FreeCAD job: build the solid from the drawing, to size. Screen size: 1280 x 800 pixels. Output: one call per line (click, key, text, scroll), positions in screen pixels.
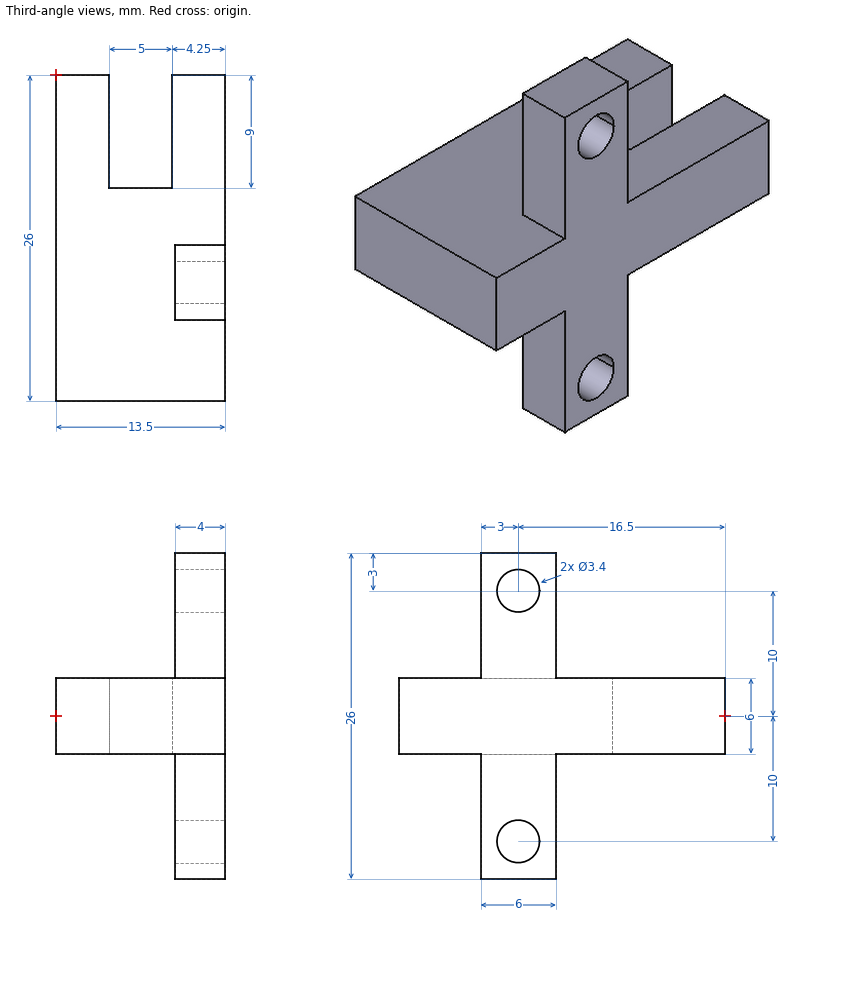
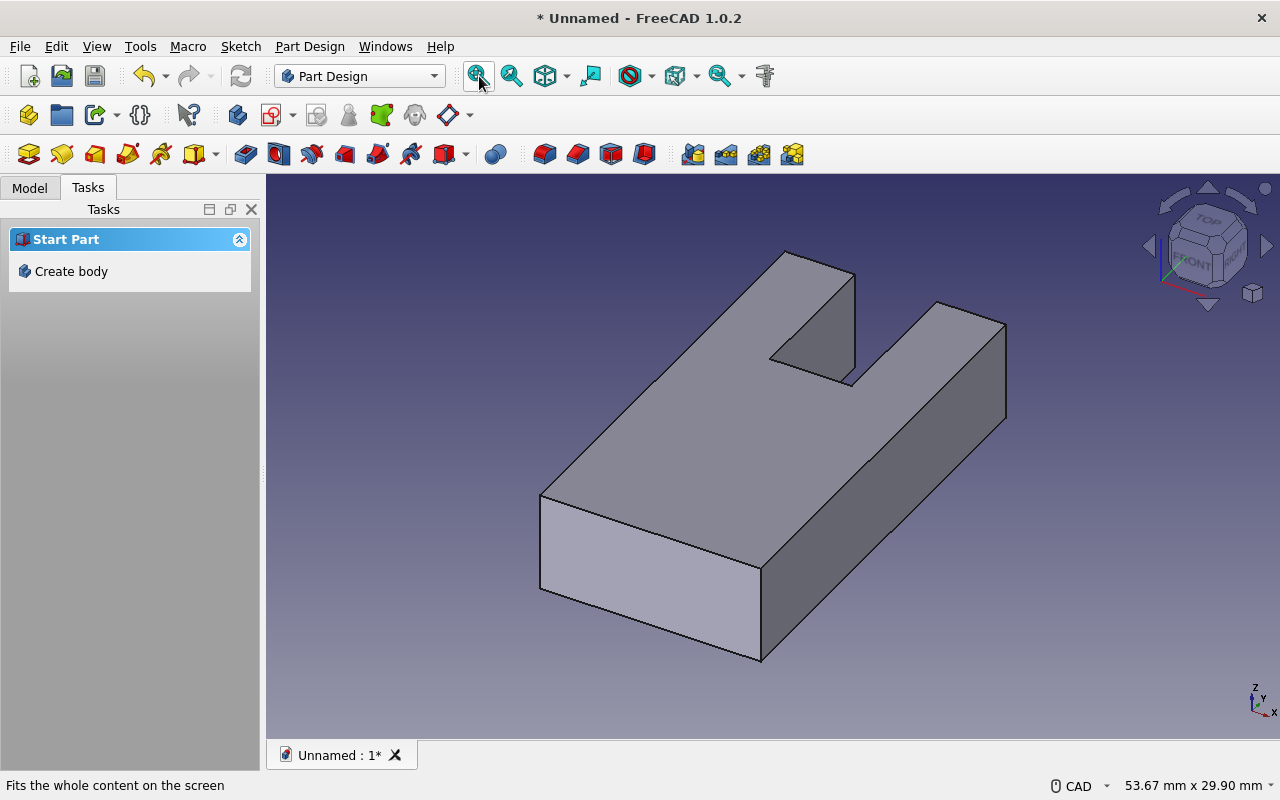
click(954, 422)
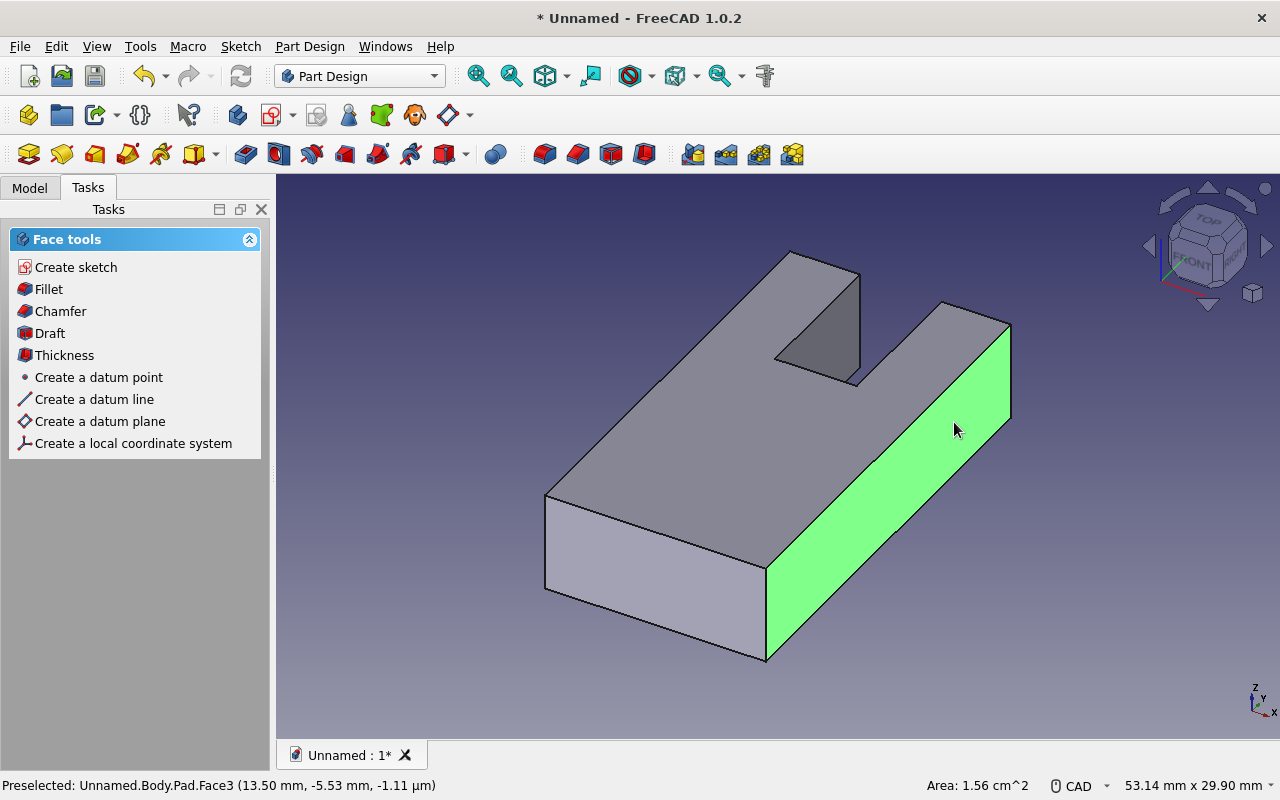
click(270, 116)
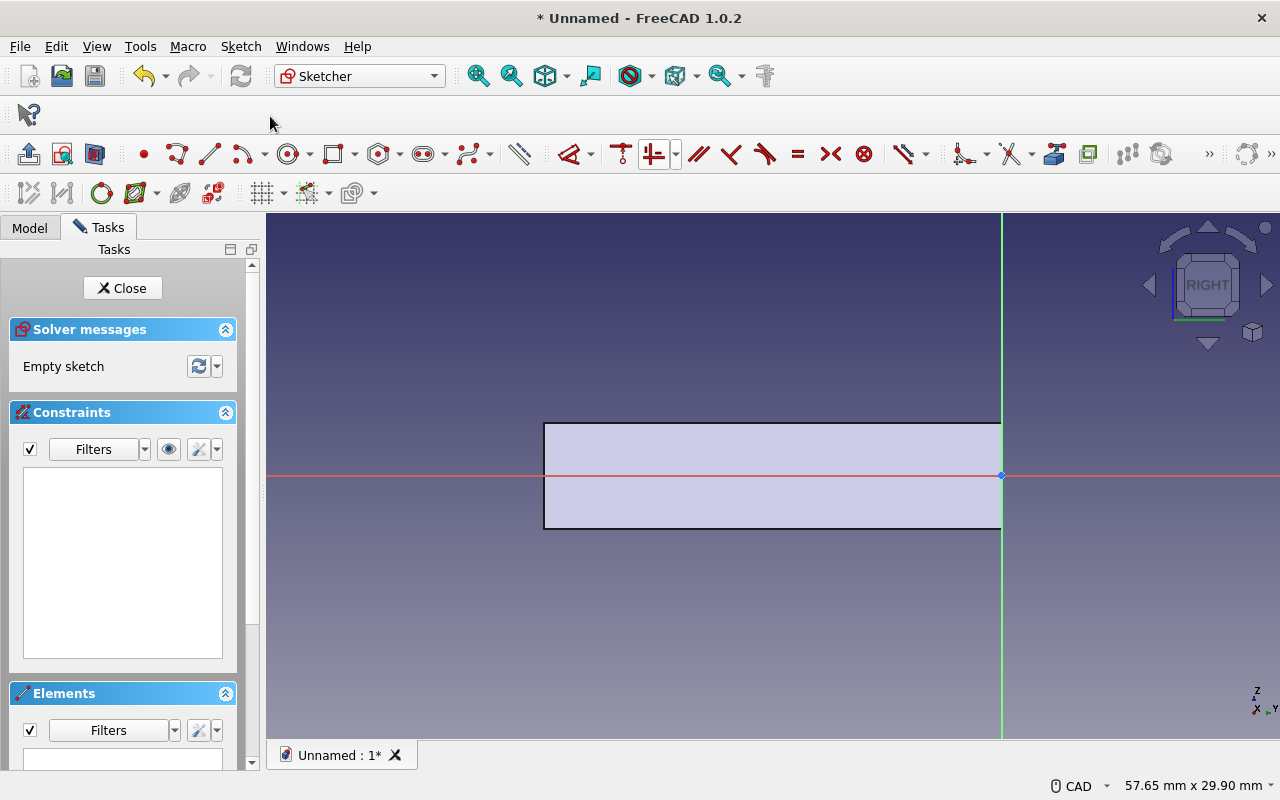
scroll(449, 476, down, 2)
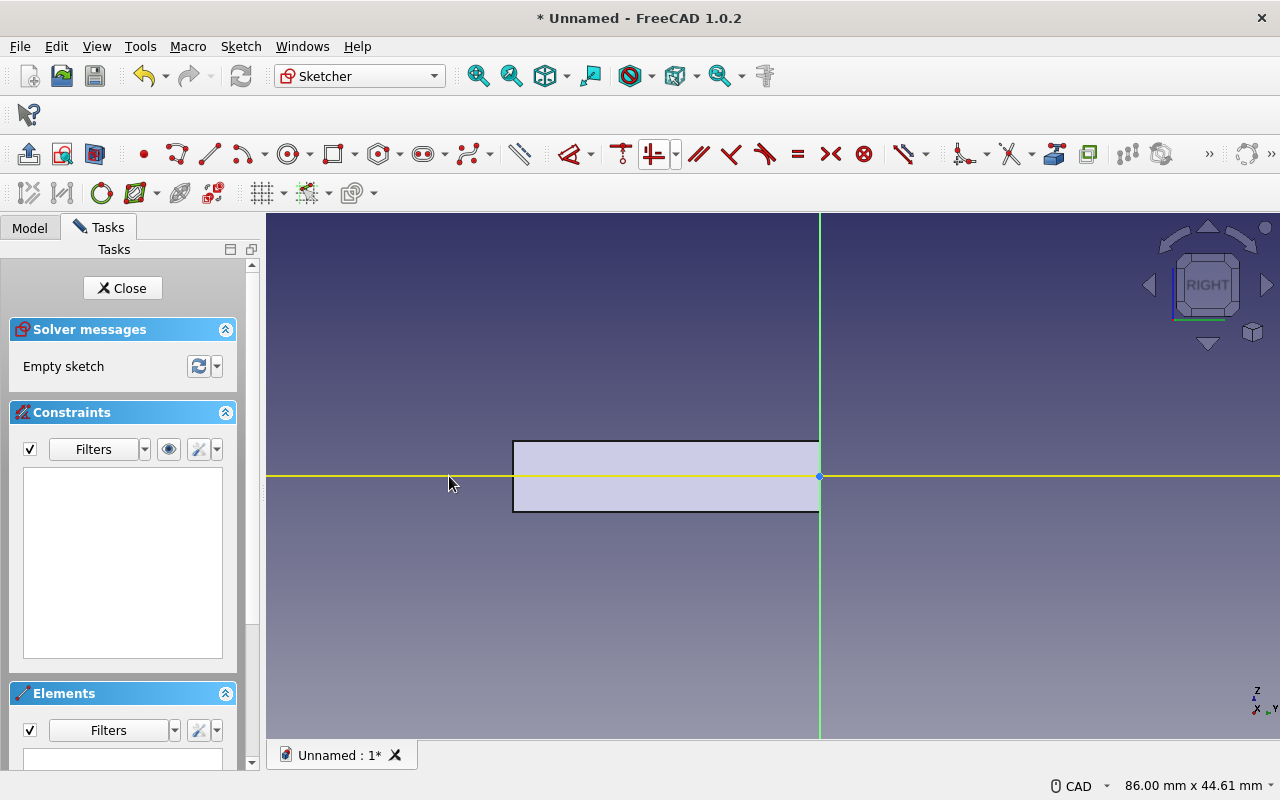
click(332, 154)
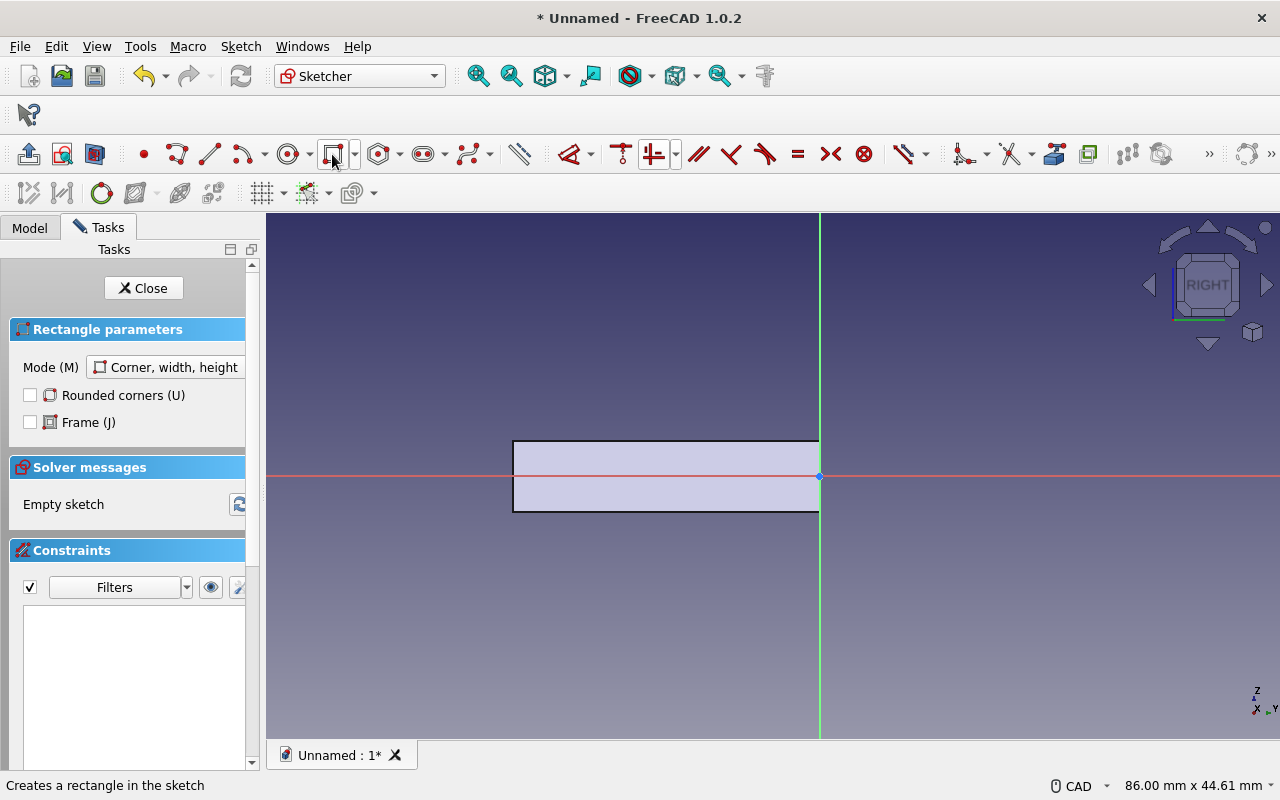
click(590, 323)
move(660, 629)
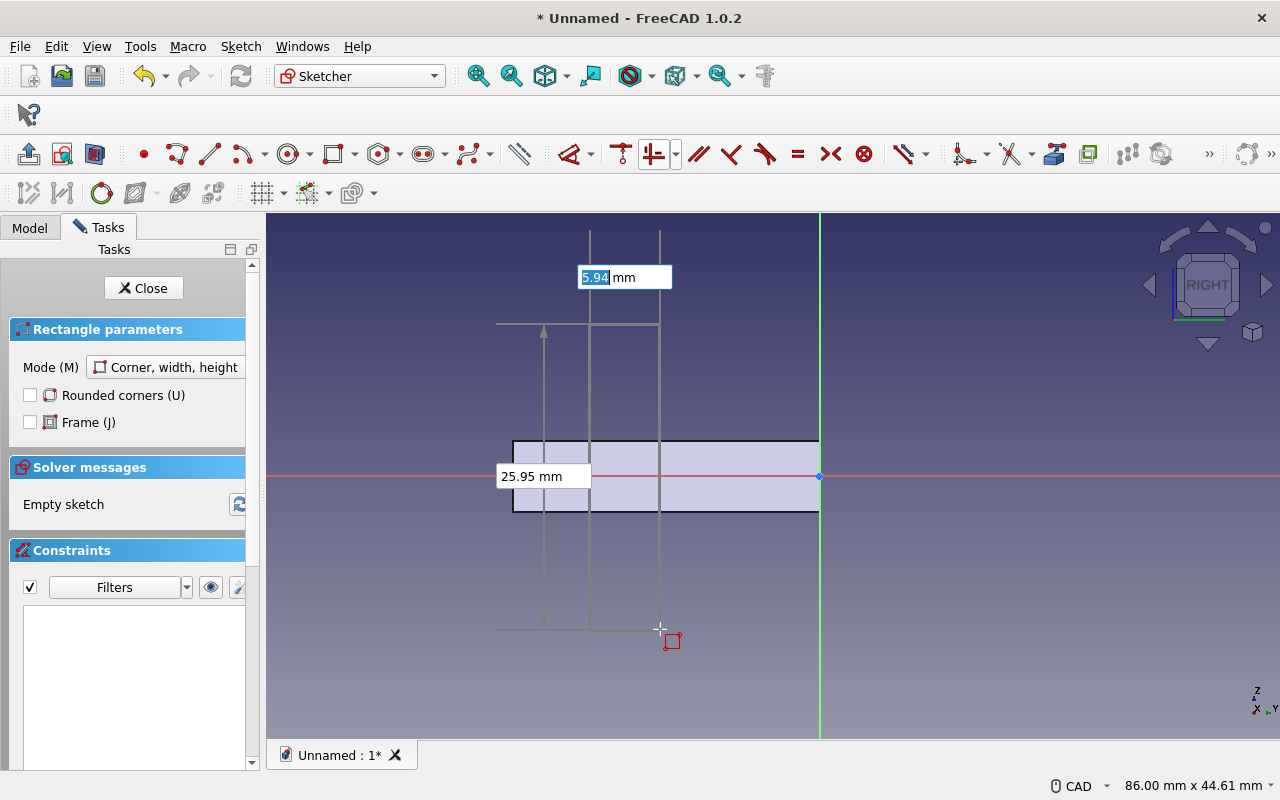
text(6)
key(Tab)
text(26)
key(Return)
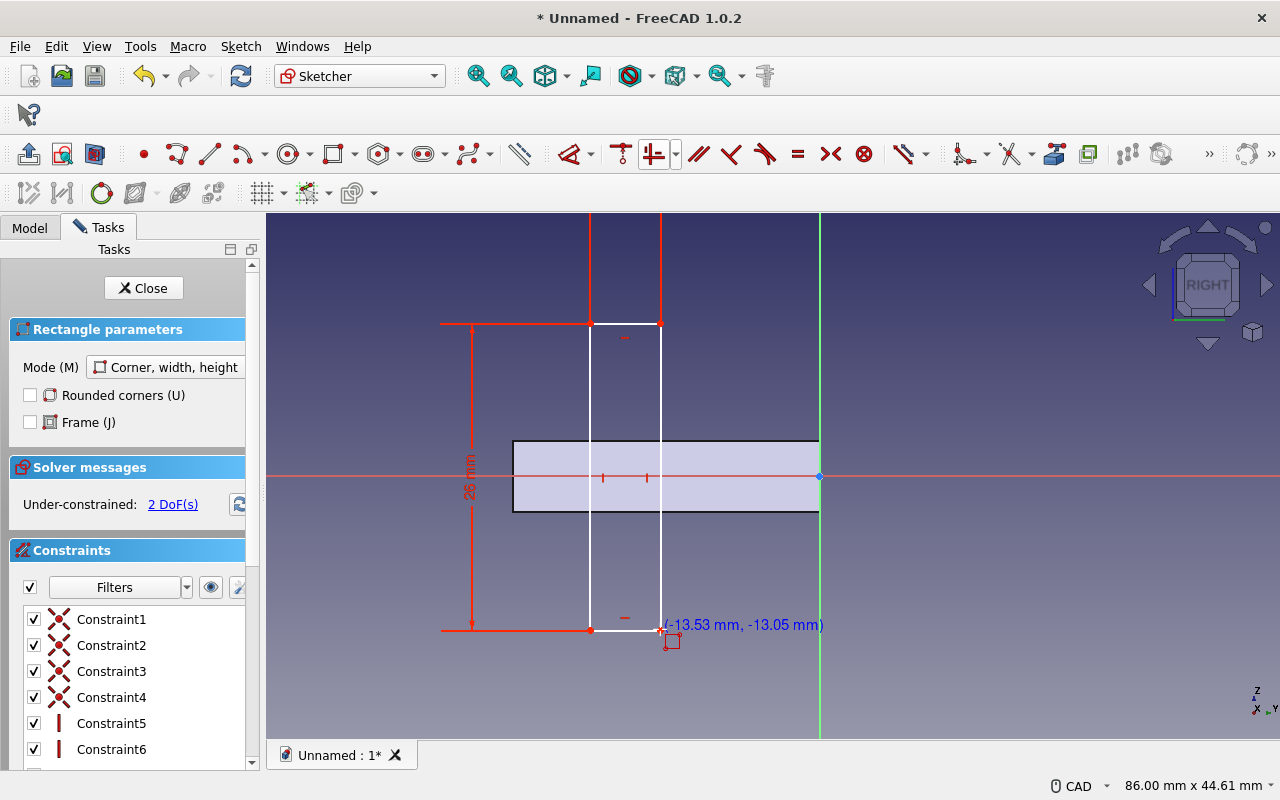
click(288, 154)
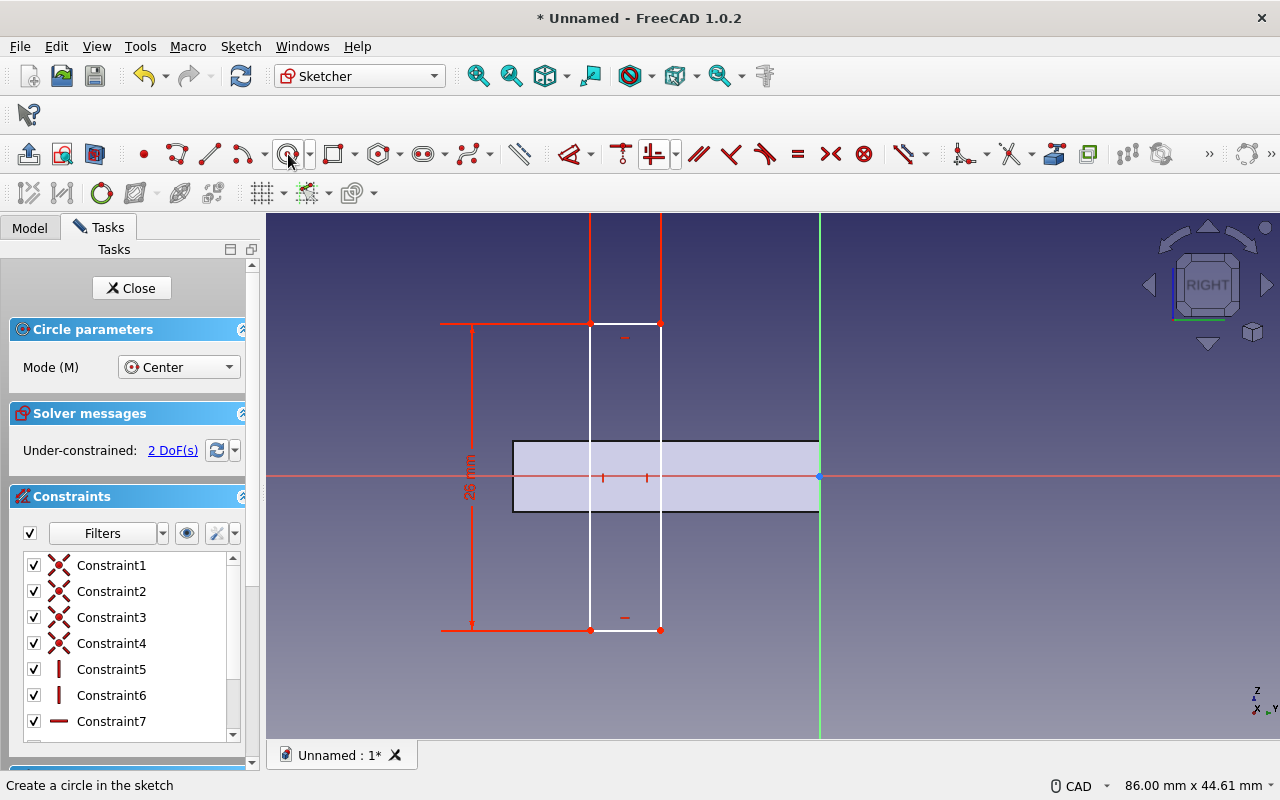
click(625, 358)
move(639, 344)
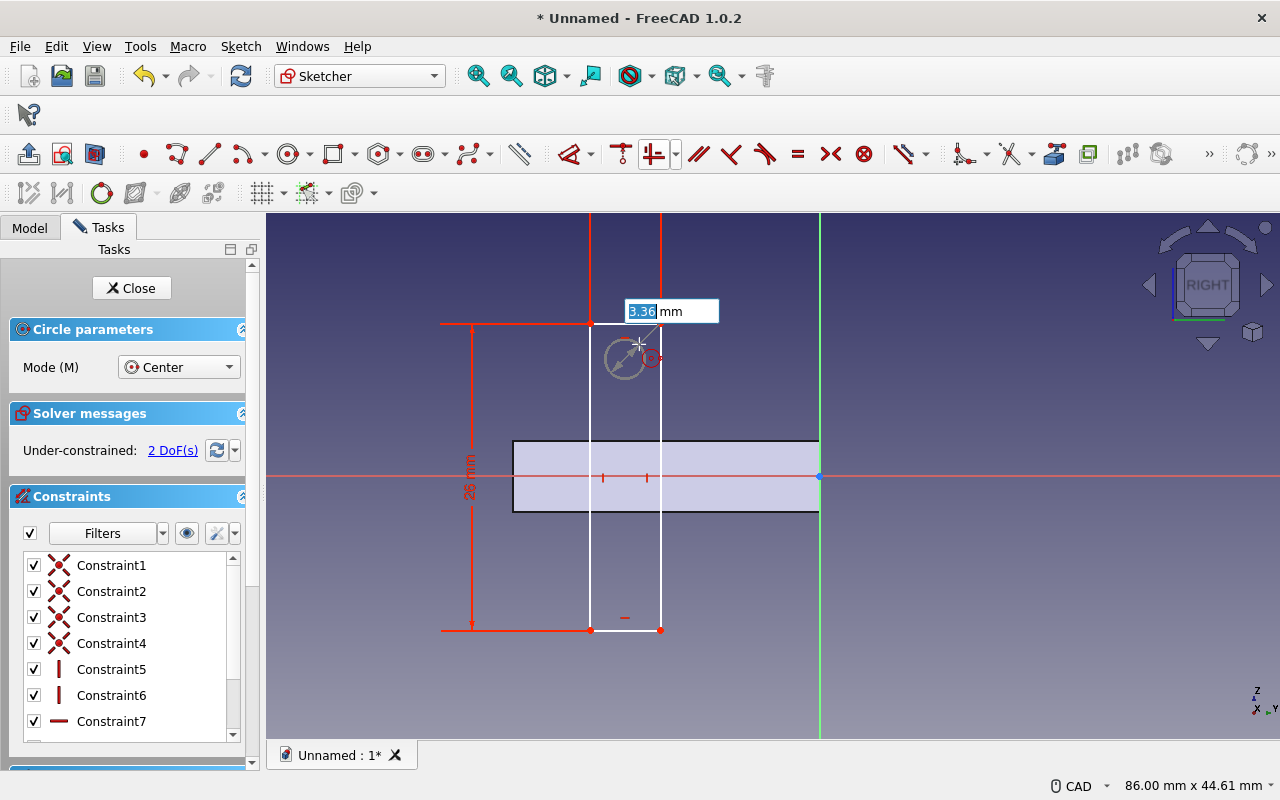
text(3.4)
key(Return)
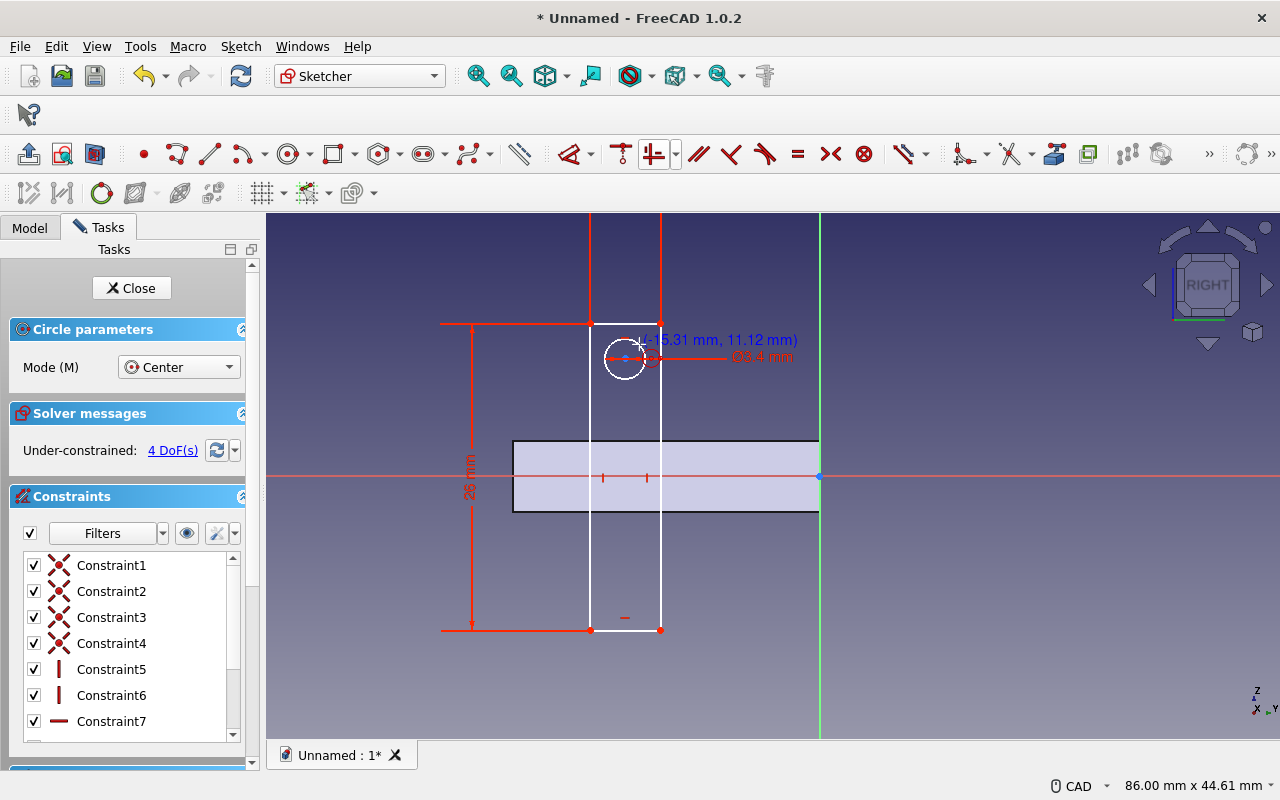
click(625, 594)
move(639, 580)